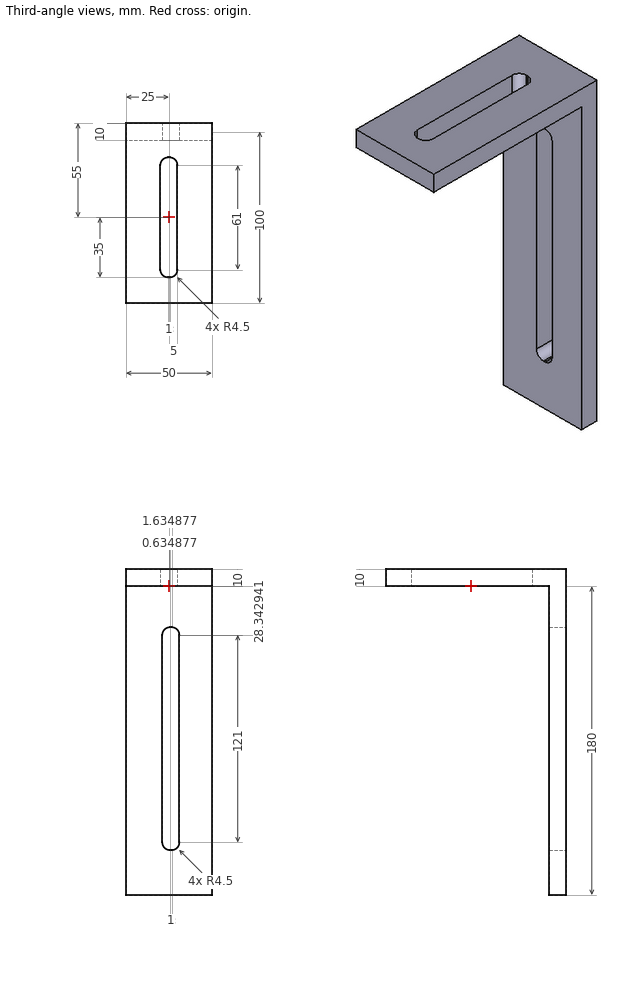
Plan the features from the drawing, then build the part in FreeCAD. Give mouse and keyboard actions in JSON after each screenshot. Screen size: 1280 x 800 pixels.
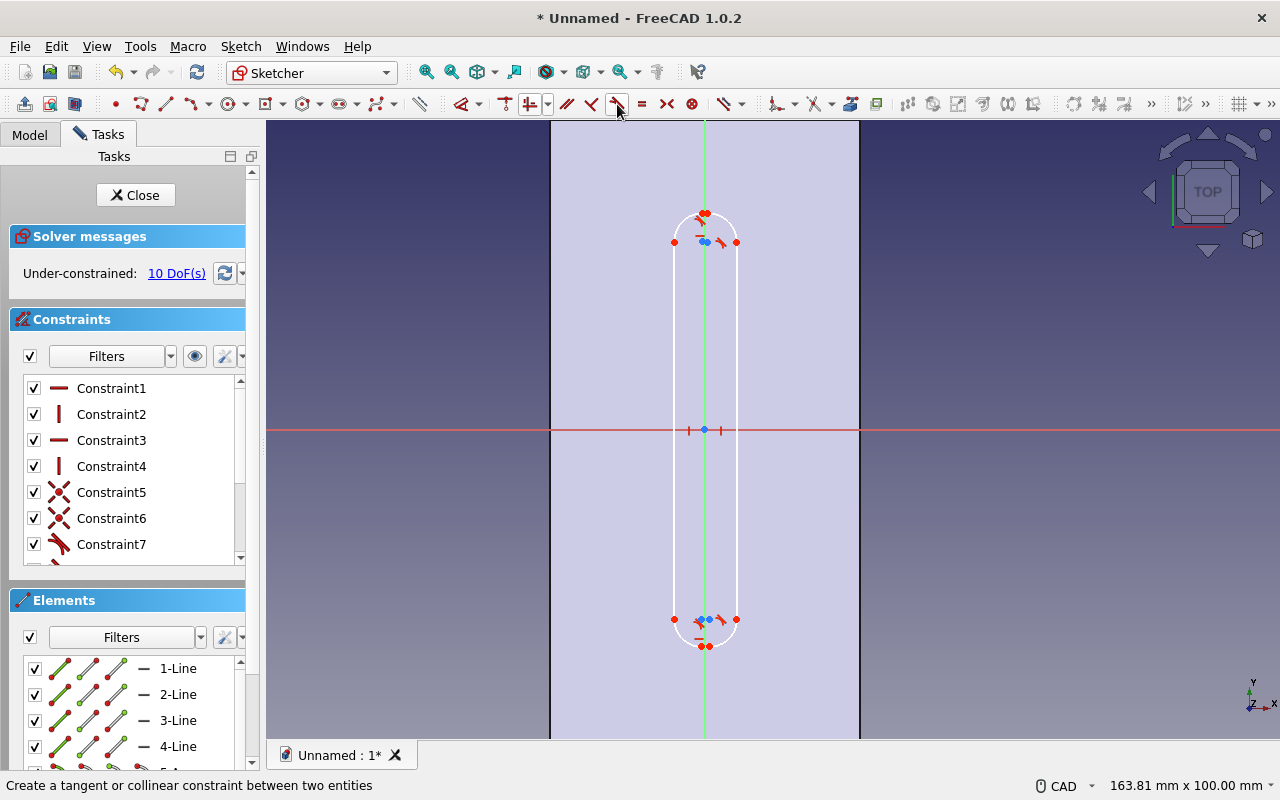
{"action": "left_click", "coordinate": [674, 356]}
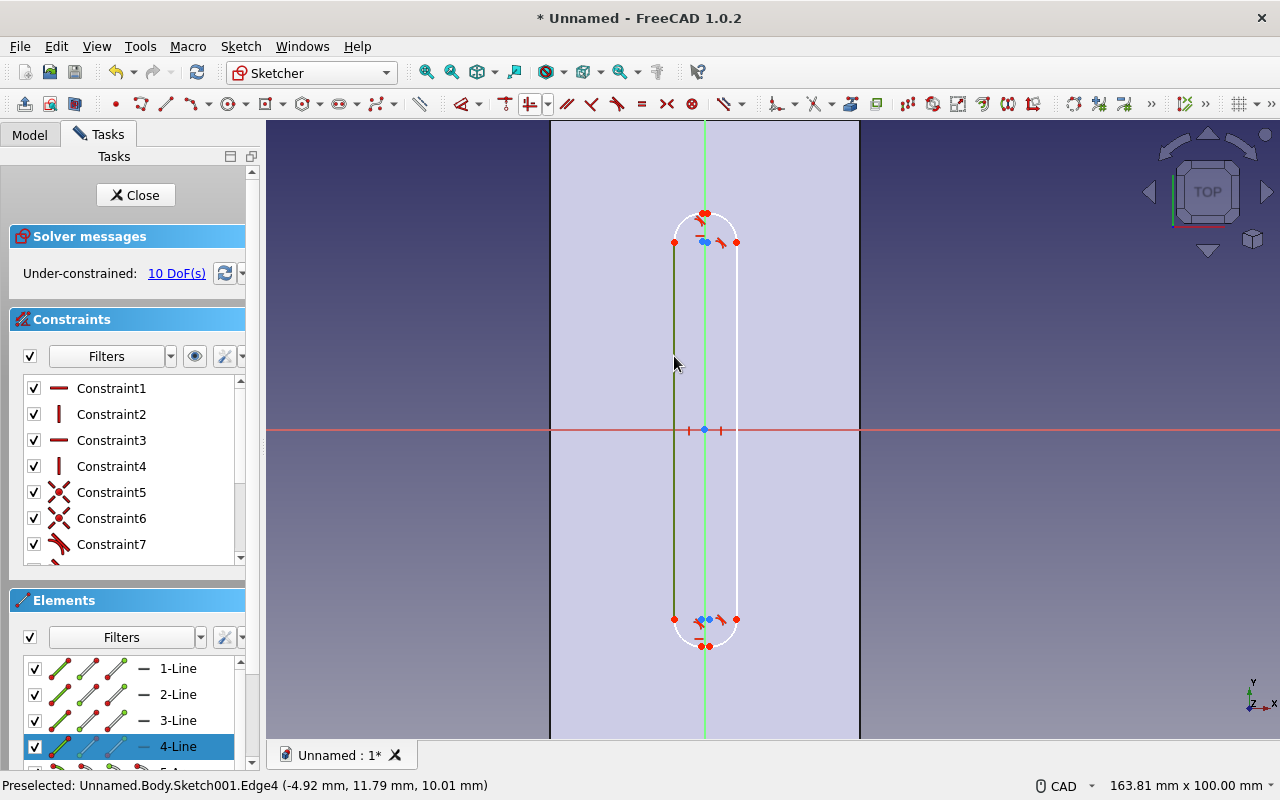
{"action": "left_click", "coordinate": [689, 217]}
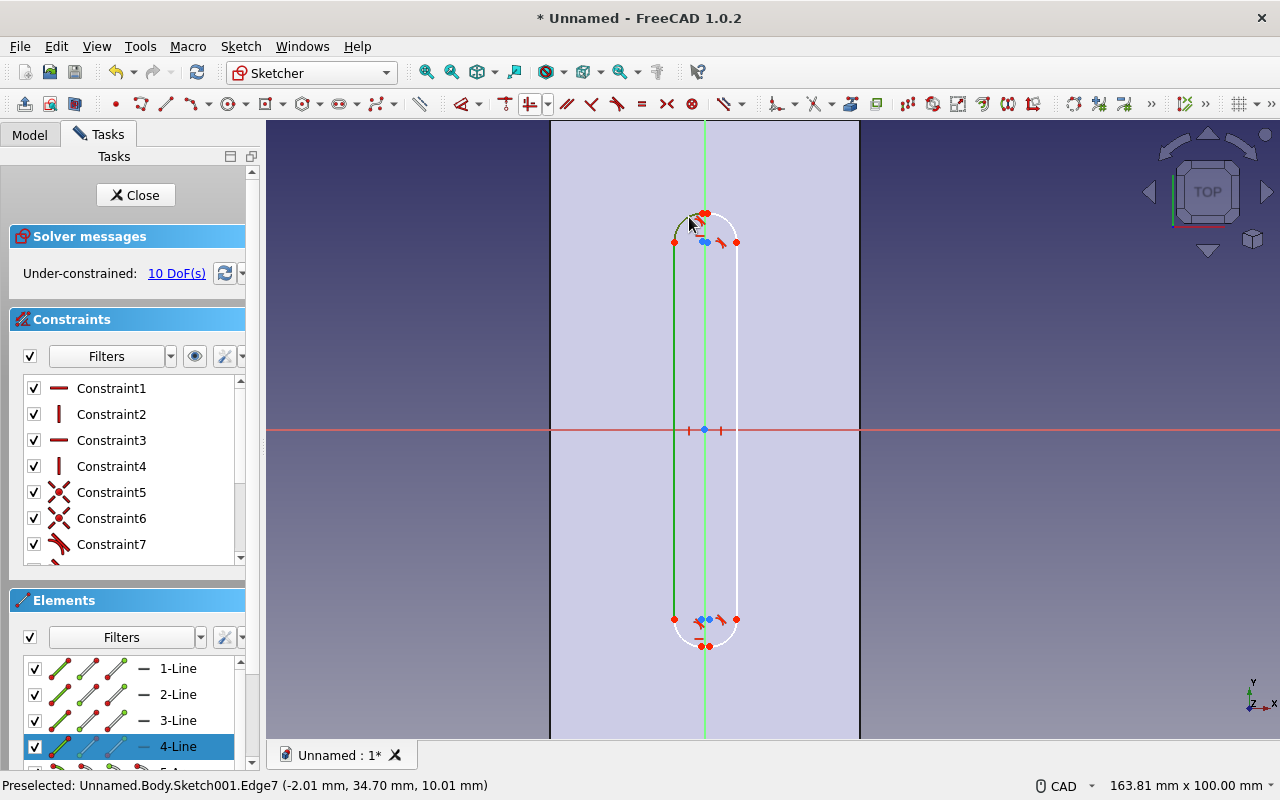
{"action": "left_click", "coordinate": [617, 104]}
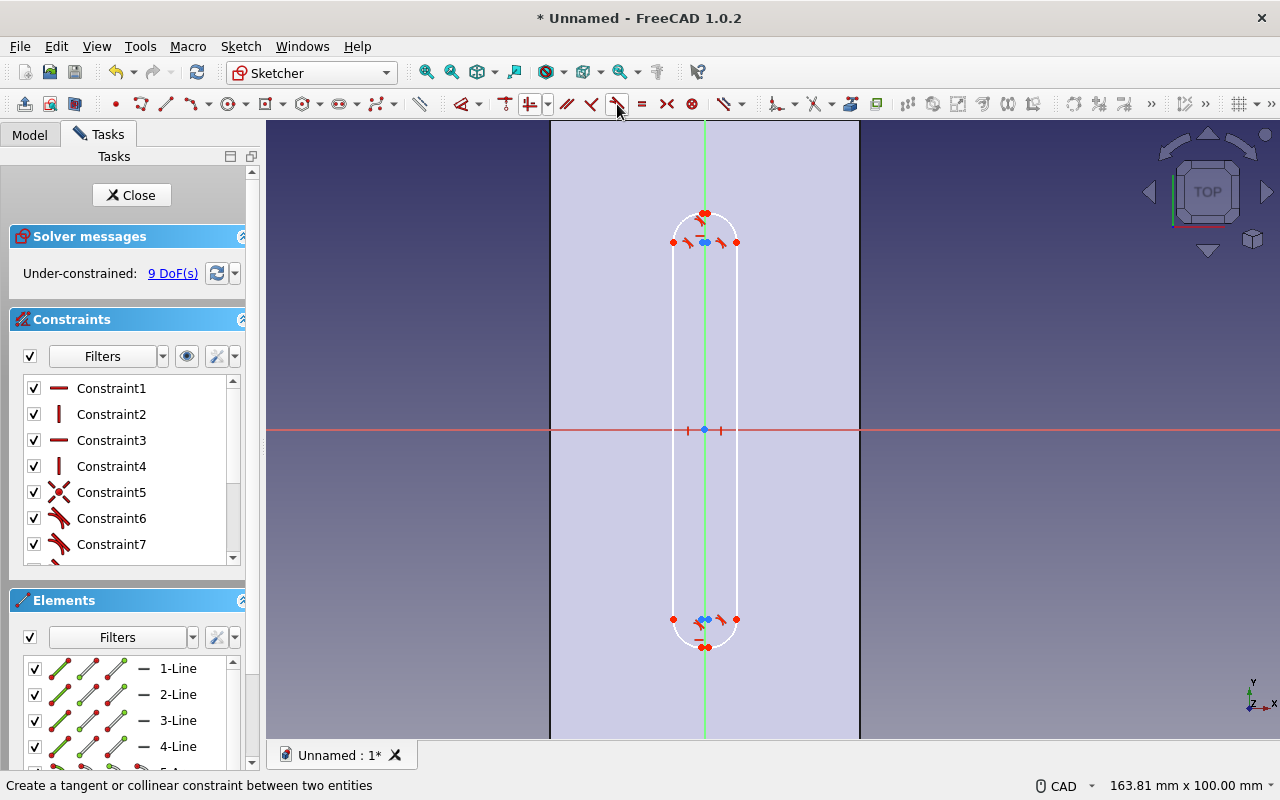
{"action": "left_click", "coordinate": [673, 356]}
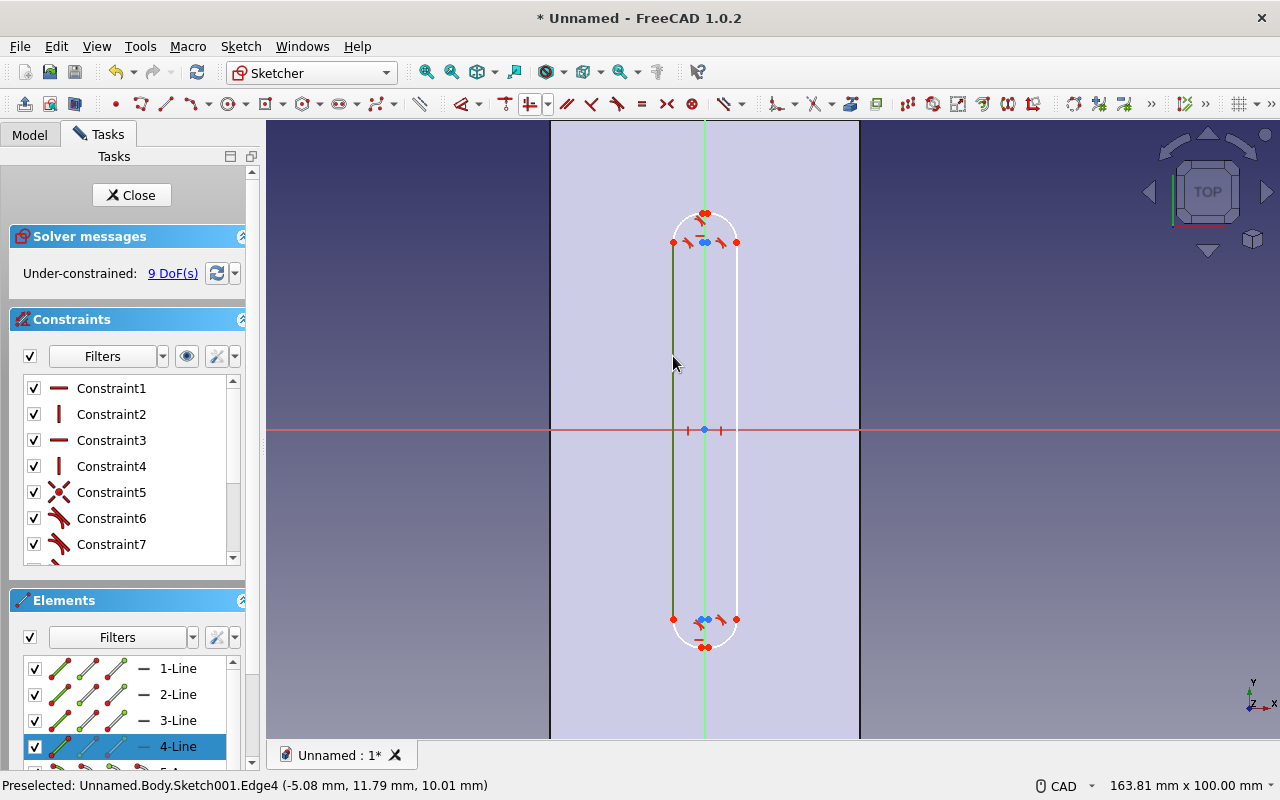
{"action": "left_click", "coordinate": [677, 632]}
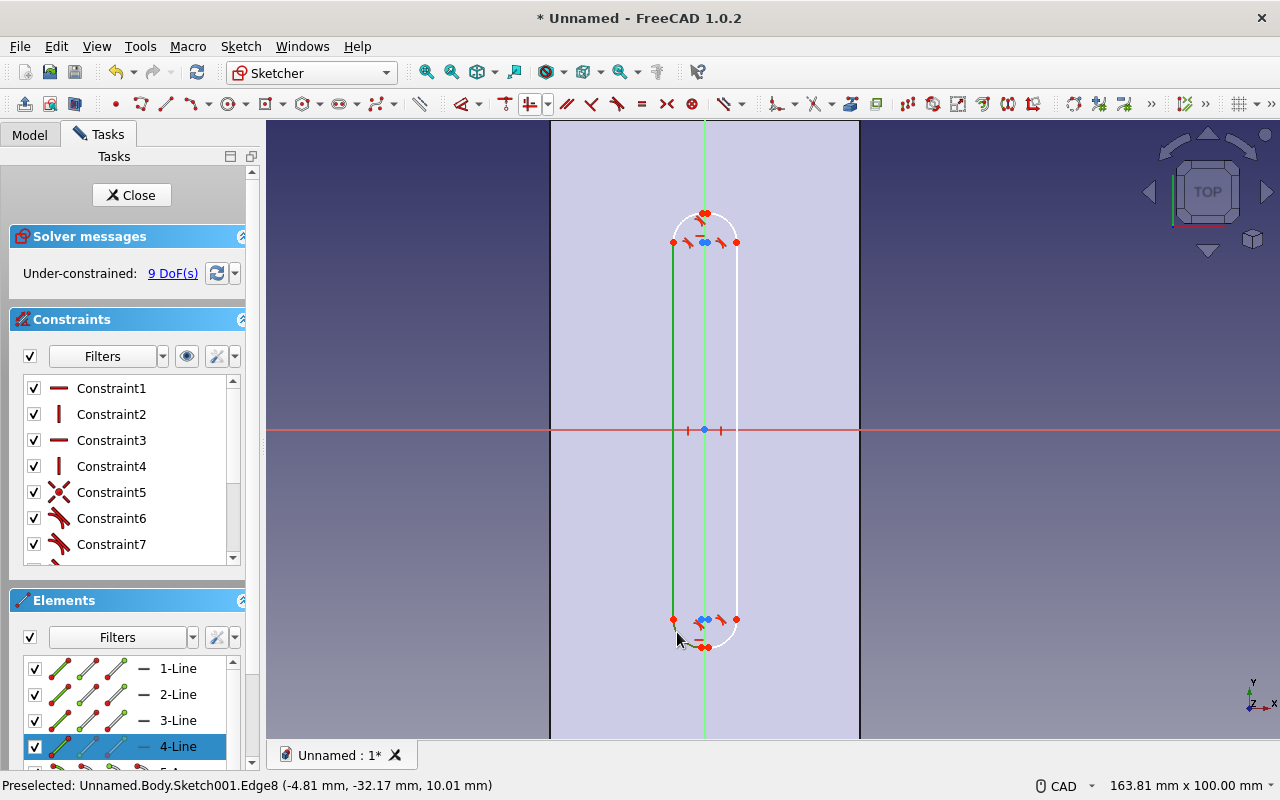
{"action": "left_click", "coordinate": [617, 104]}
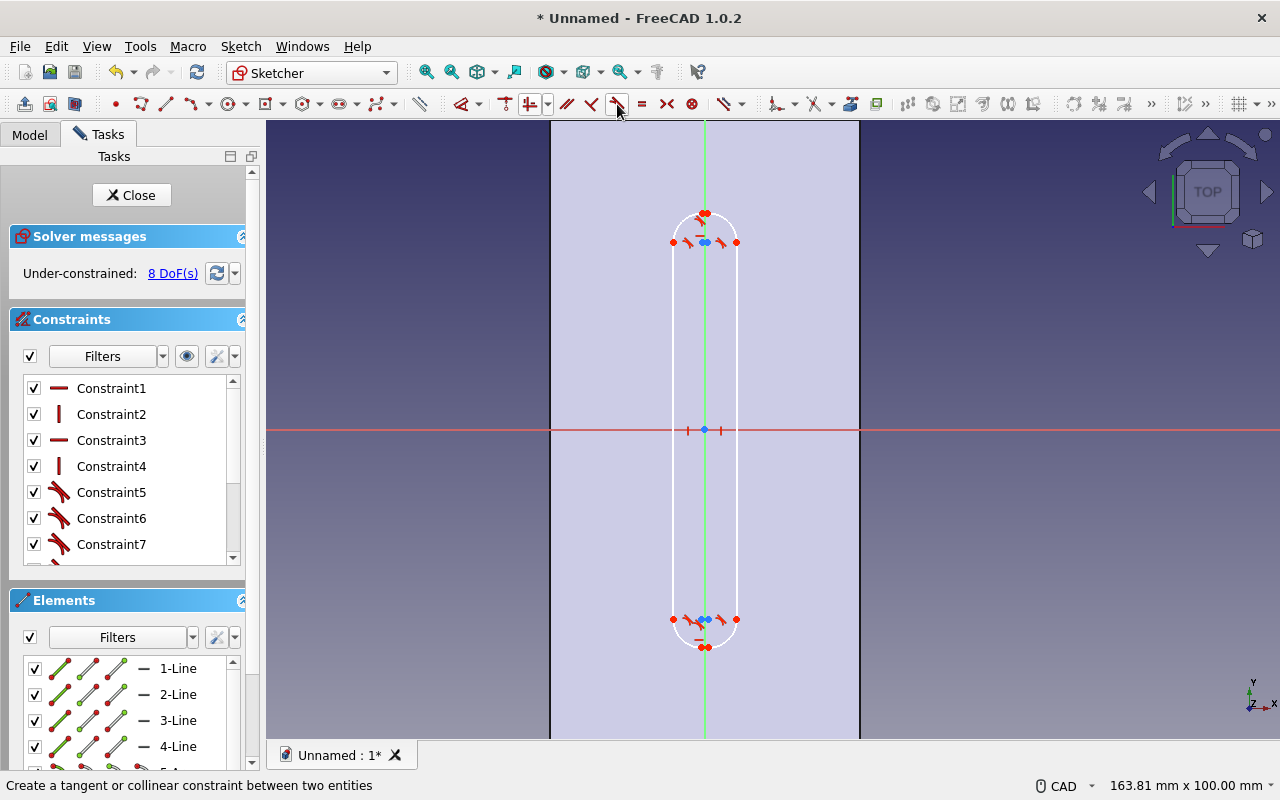
{"action": "left_click", "coordinate": [721, 645]}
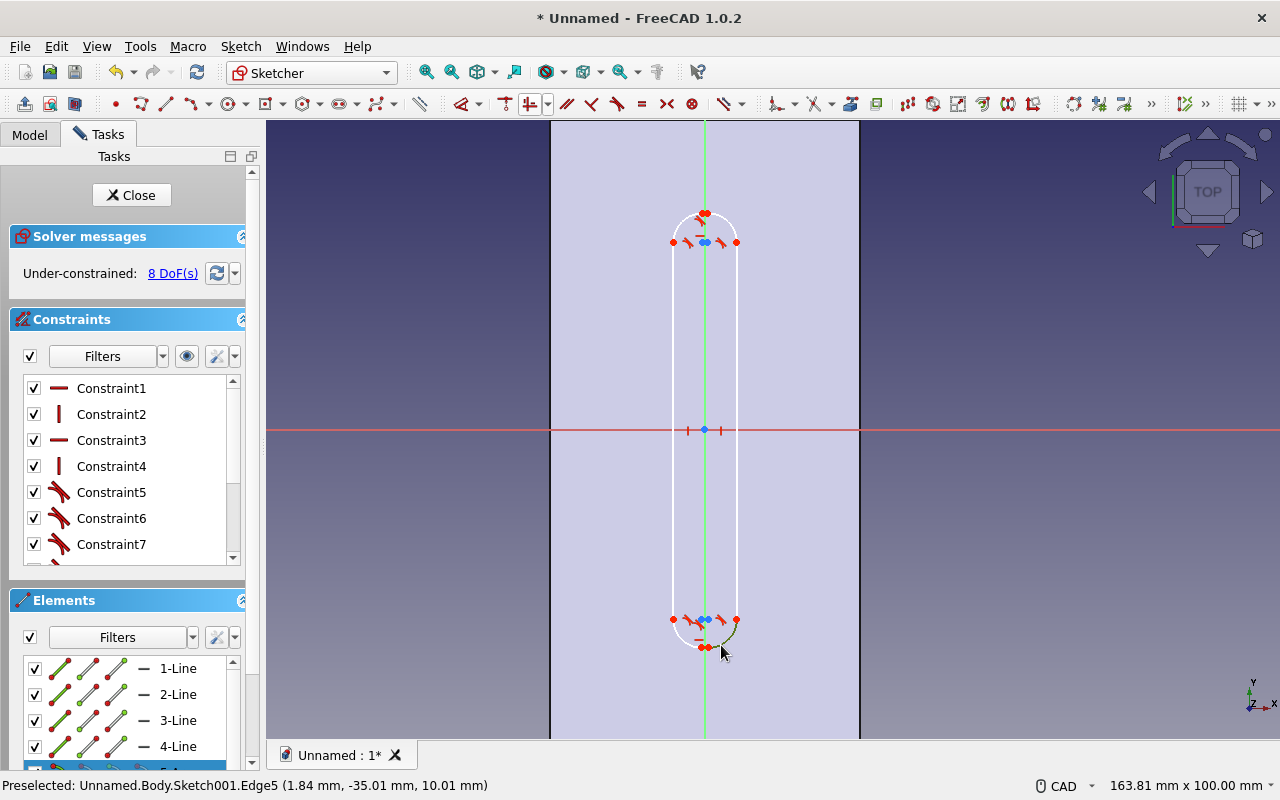
{"action": "left_click", "coordinate": [734, 229]}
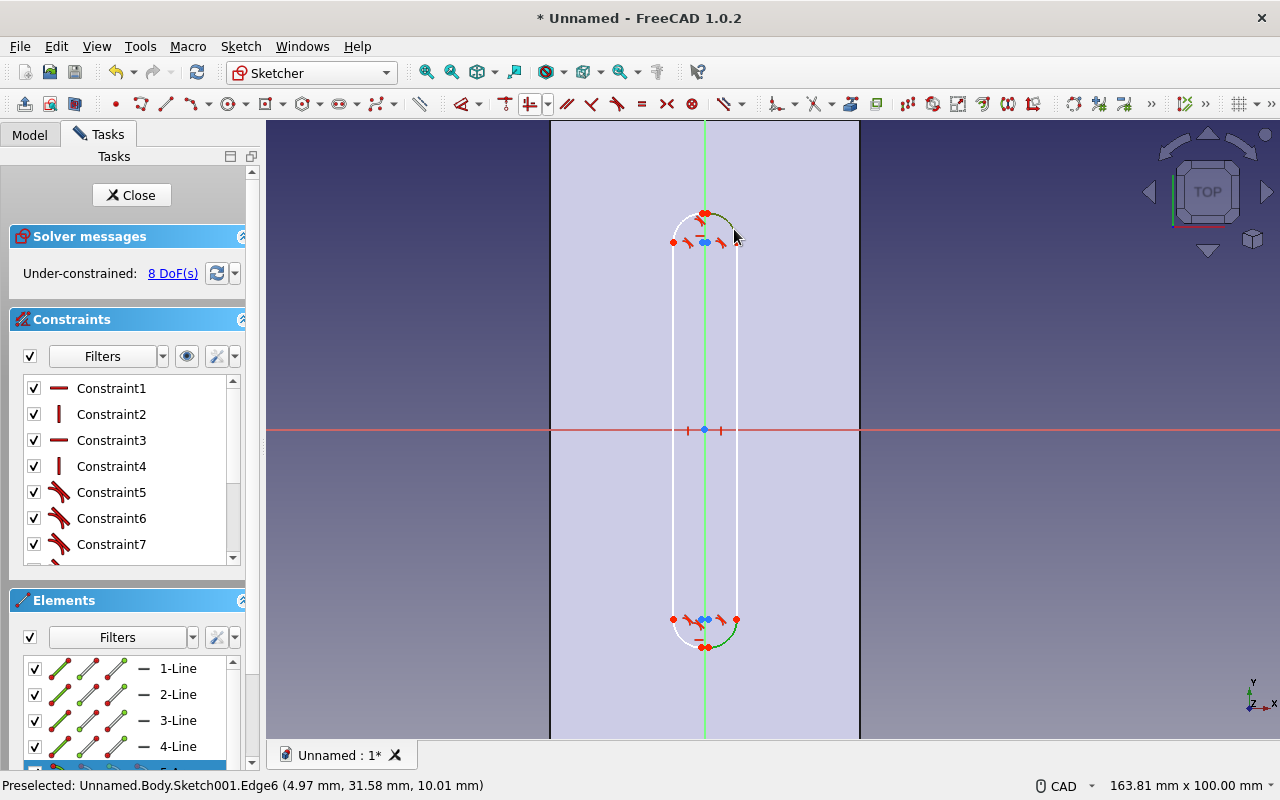
{"action": "left_click", "coordinate": [689, 217]}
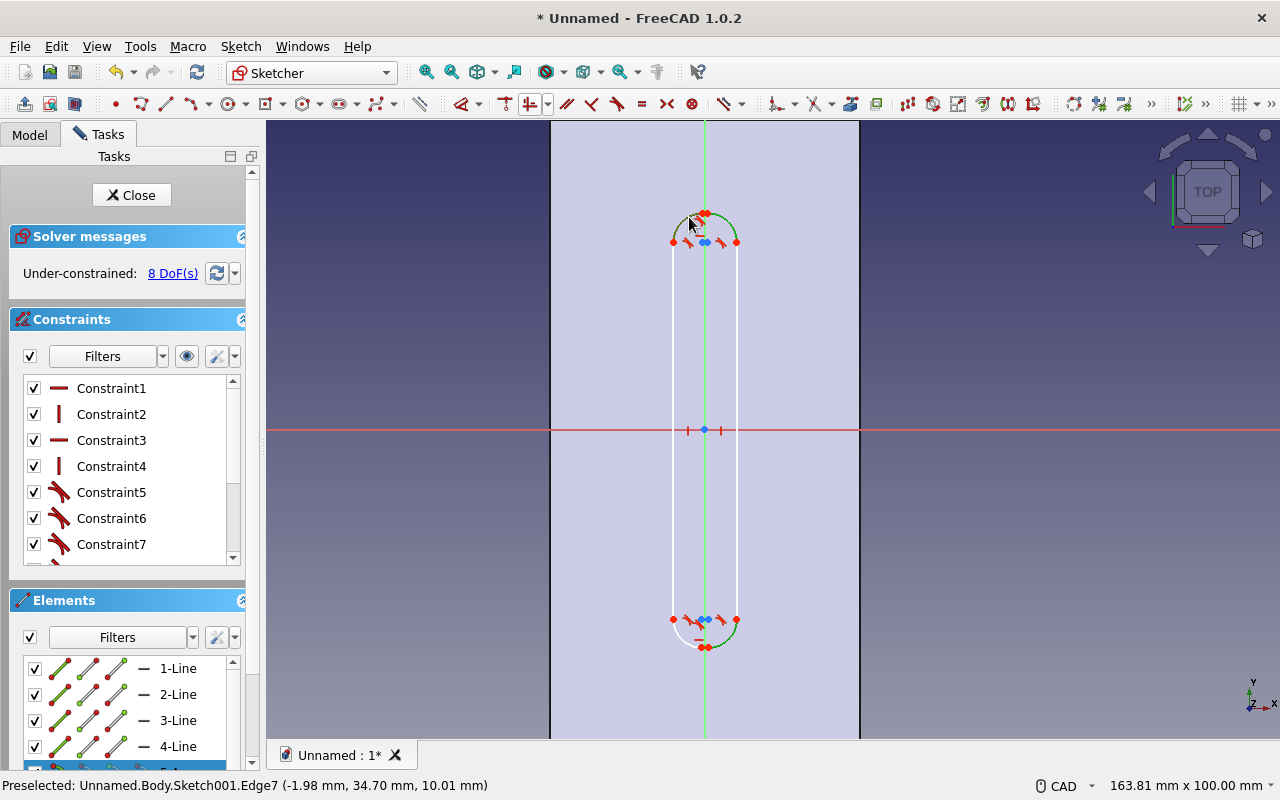
{"action": "left_click", "coordinate": [677, 632]}